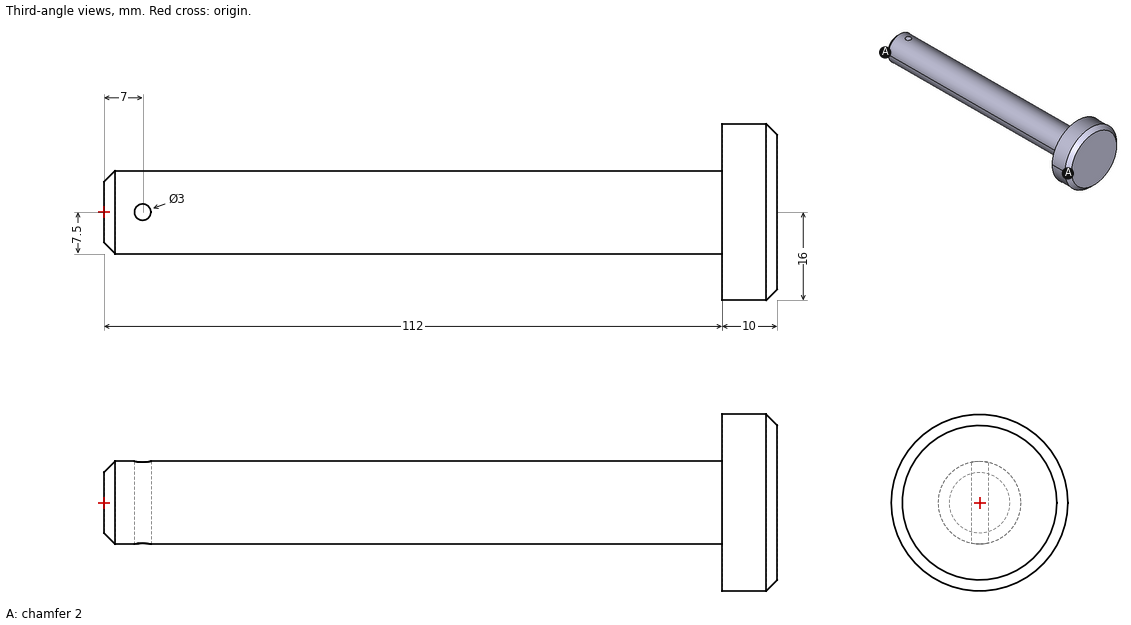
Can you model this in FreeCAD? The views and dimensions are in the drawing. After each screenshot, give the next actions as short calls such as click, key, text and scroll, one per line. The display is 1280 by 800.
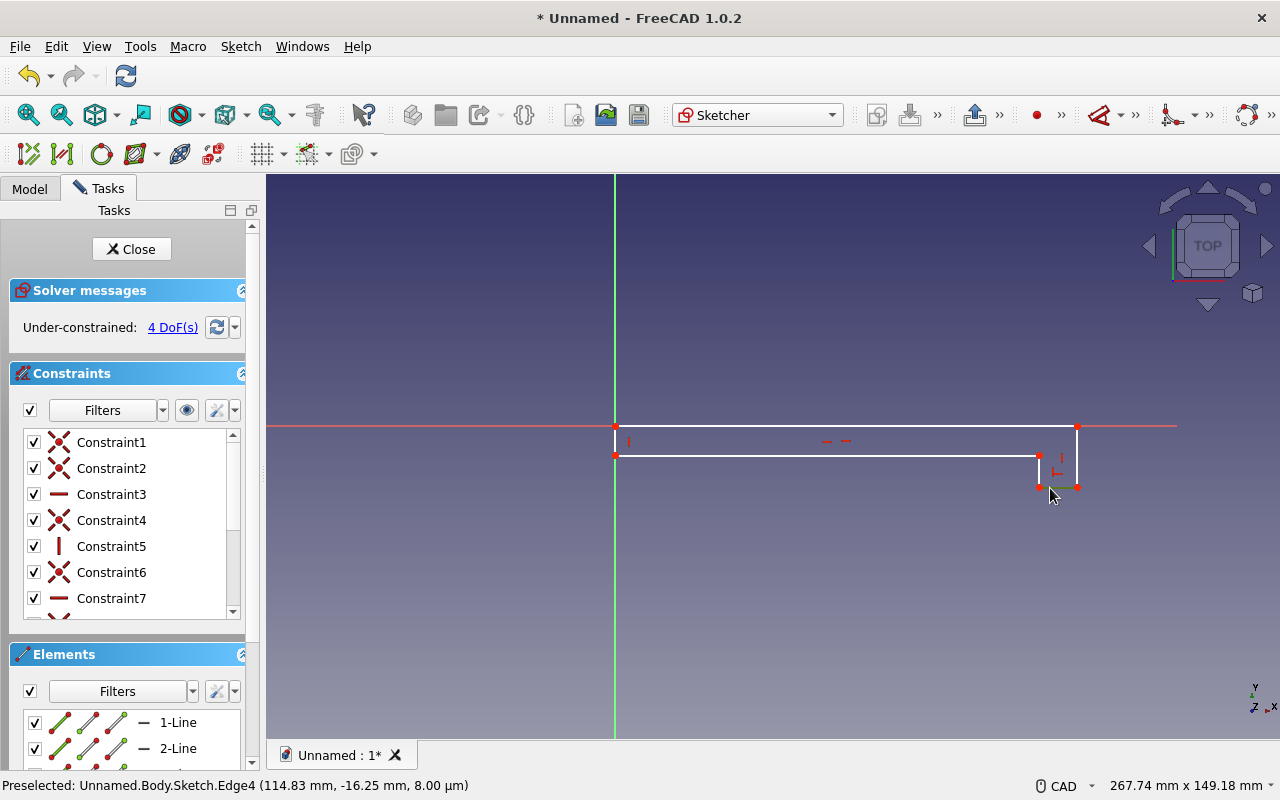
click(1120, 116)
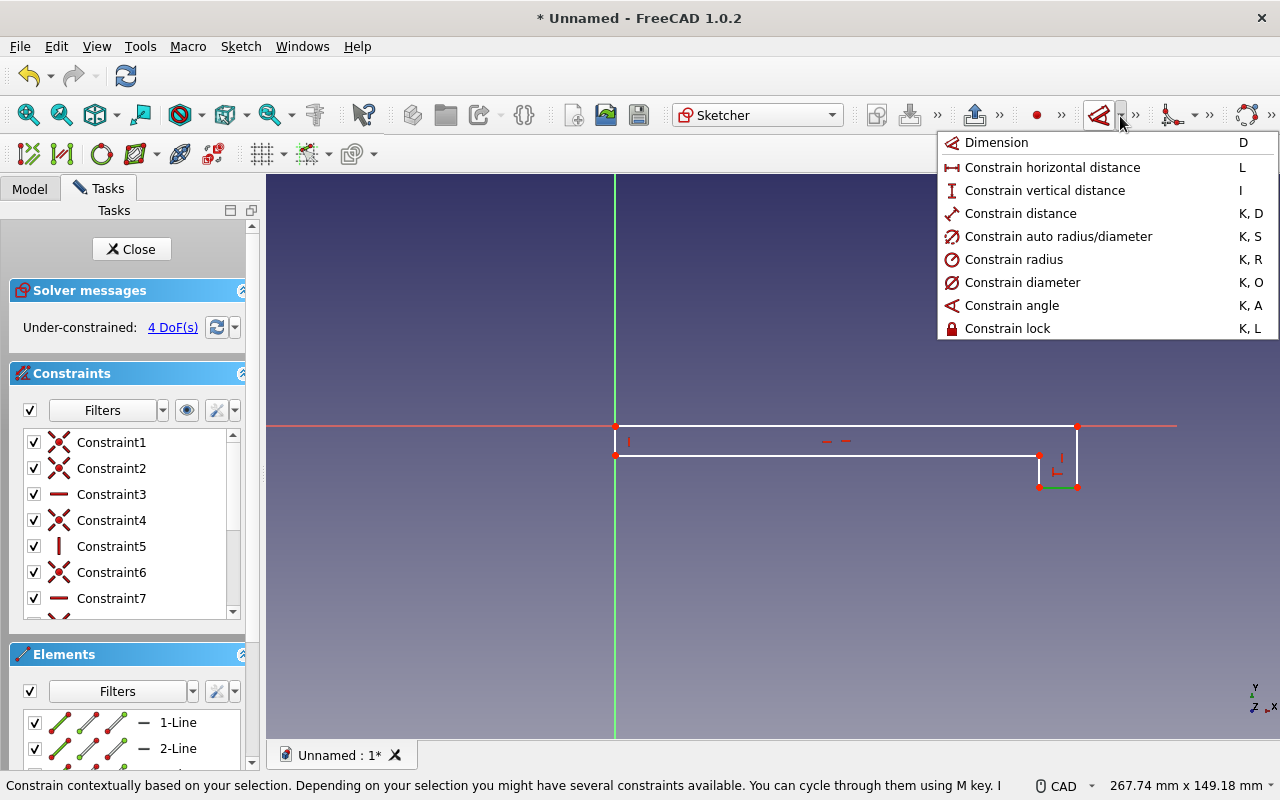
click(1108, 168)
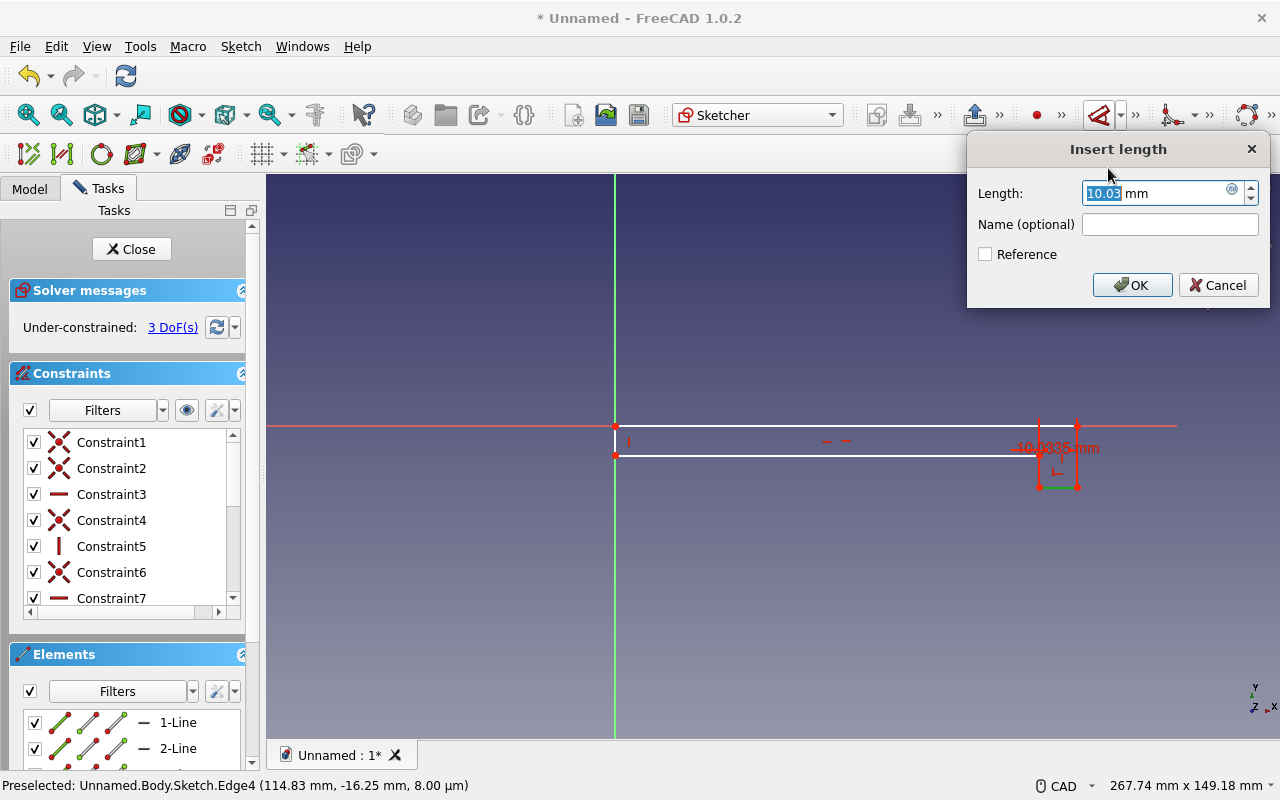
text(10)
key(Return)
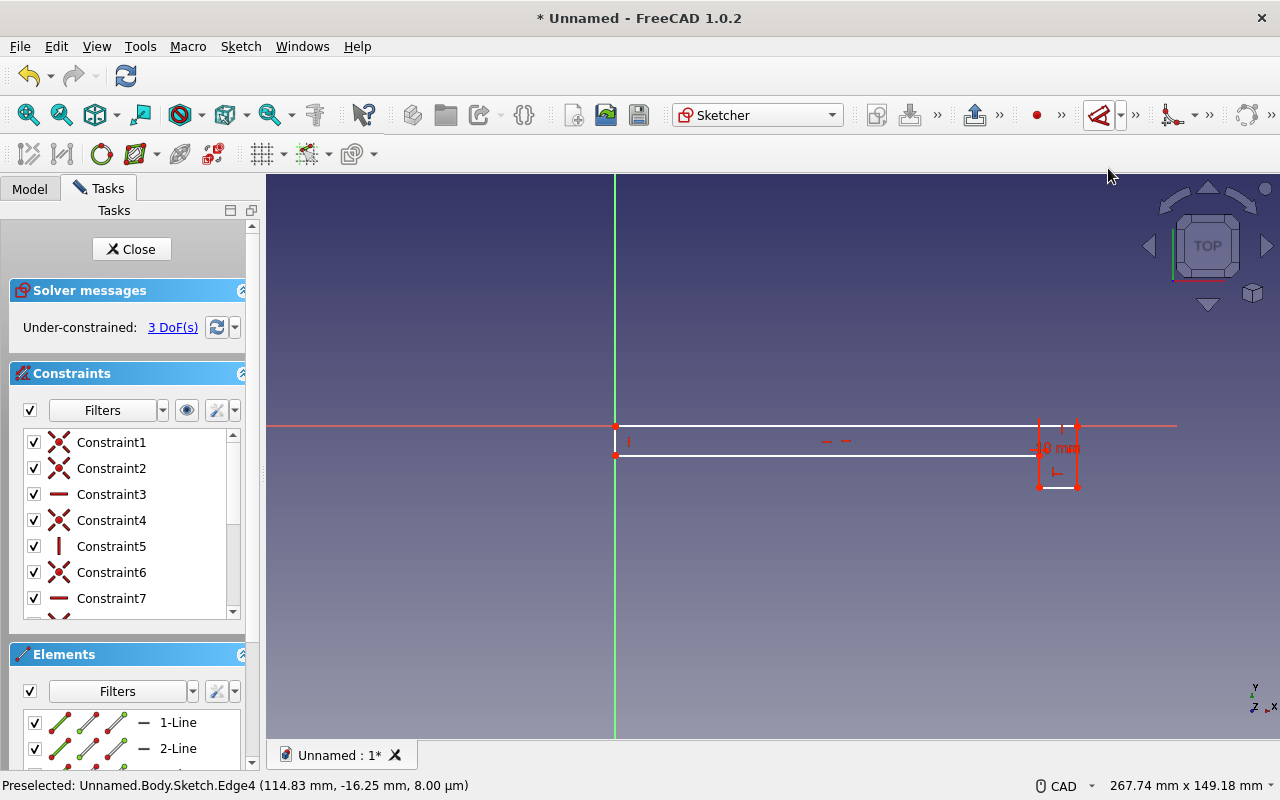
click(1077, 470)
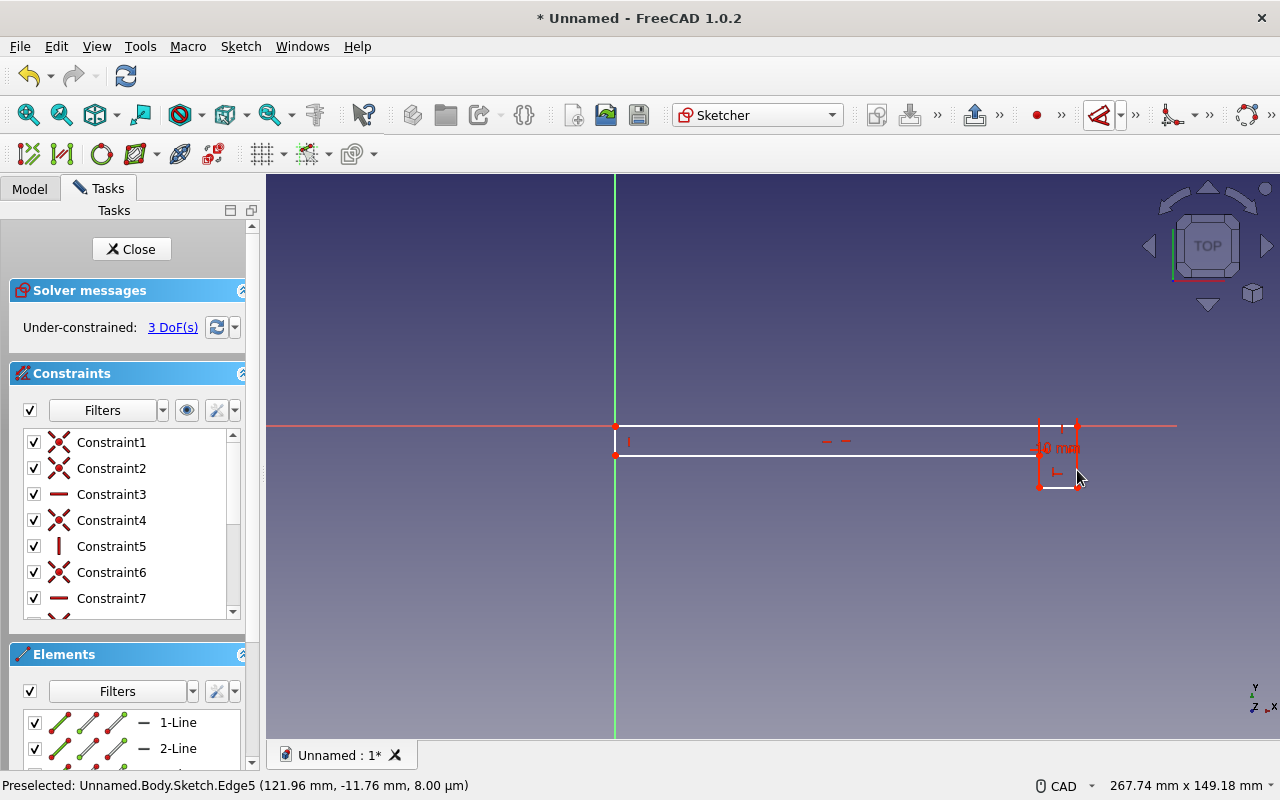
key(i)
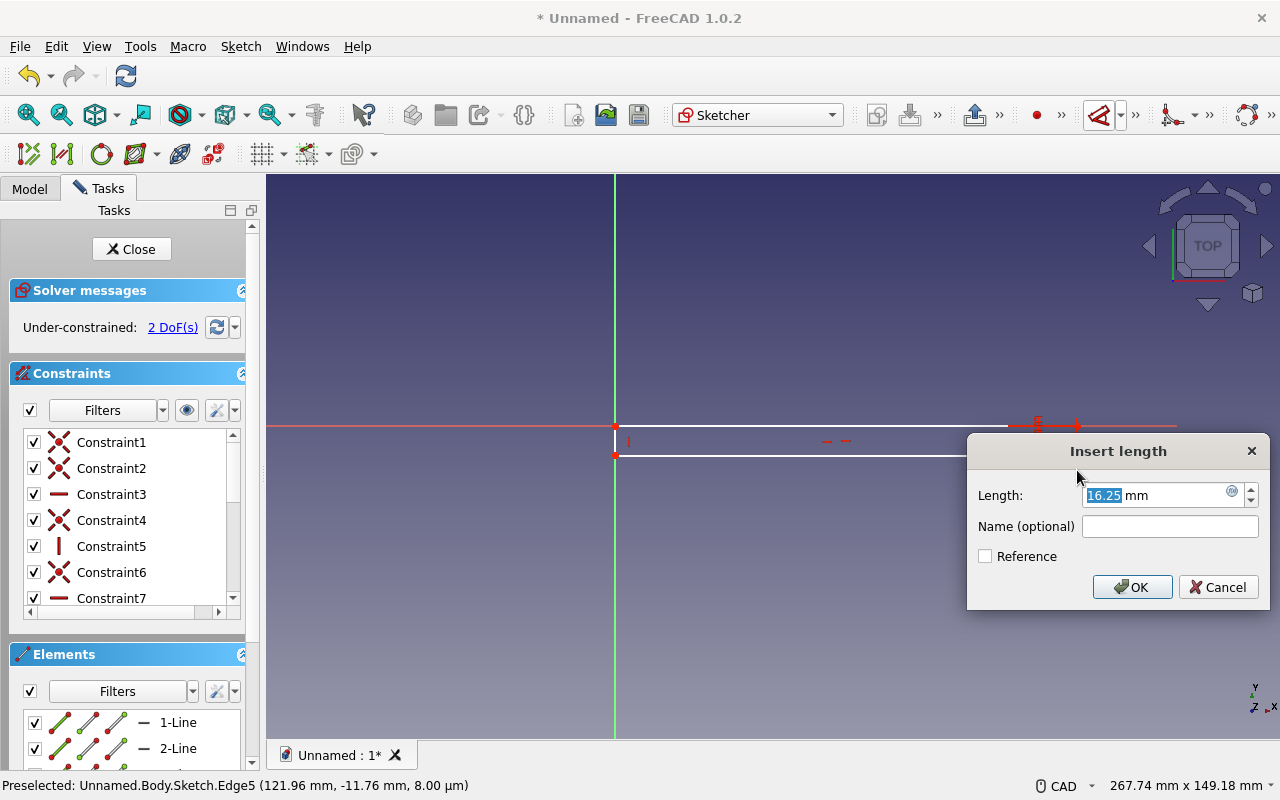
text(16)
key(Return)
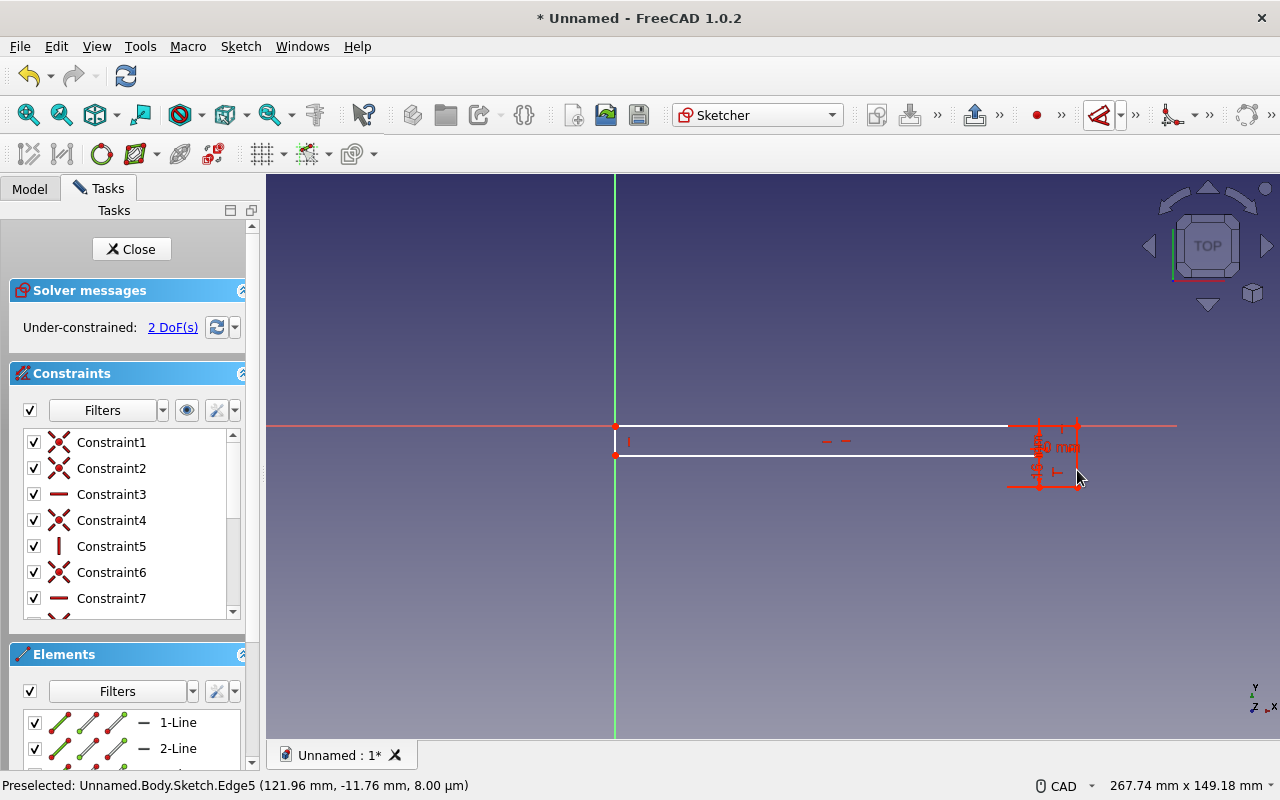
scroll(615, 438, up, 2)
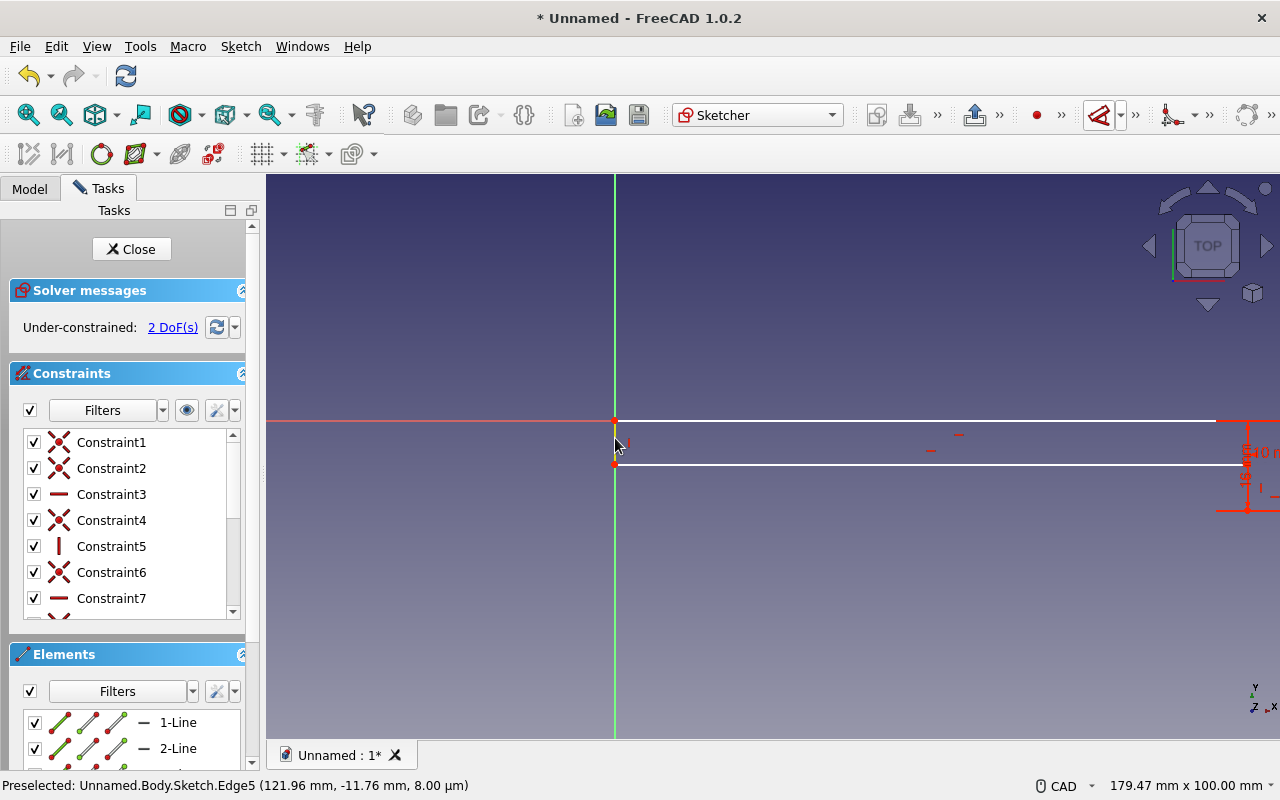
click(615, 438)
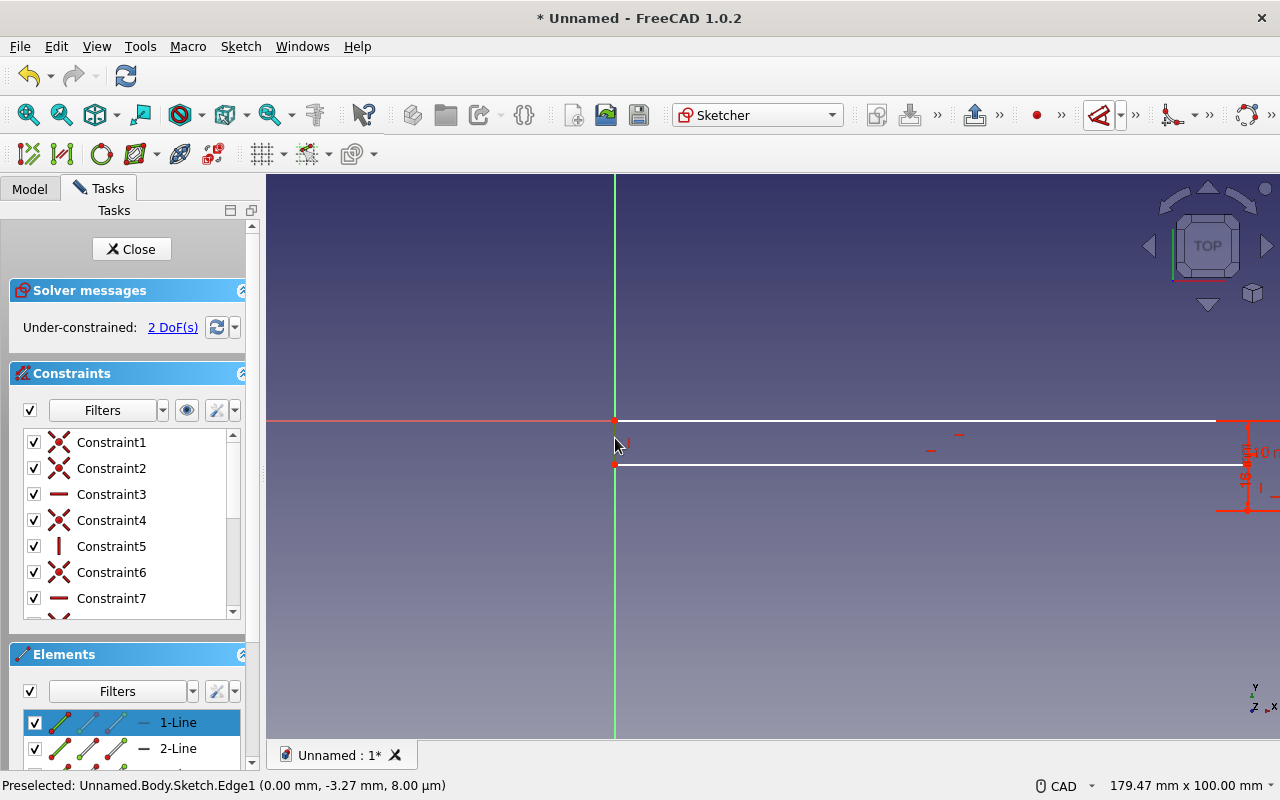
click(1120, 116)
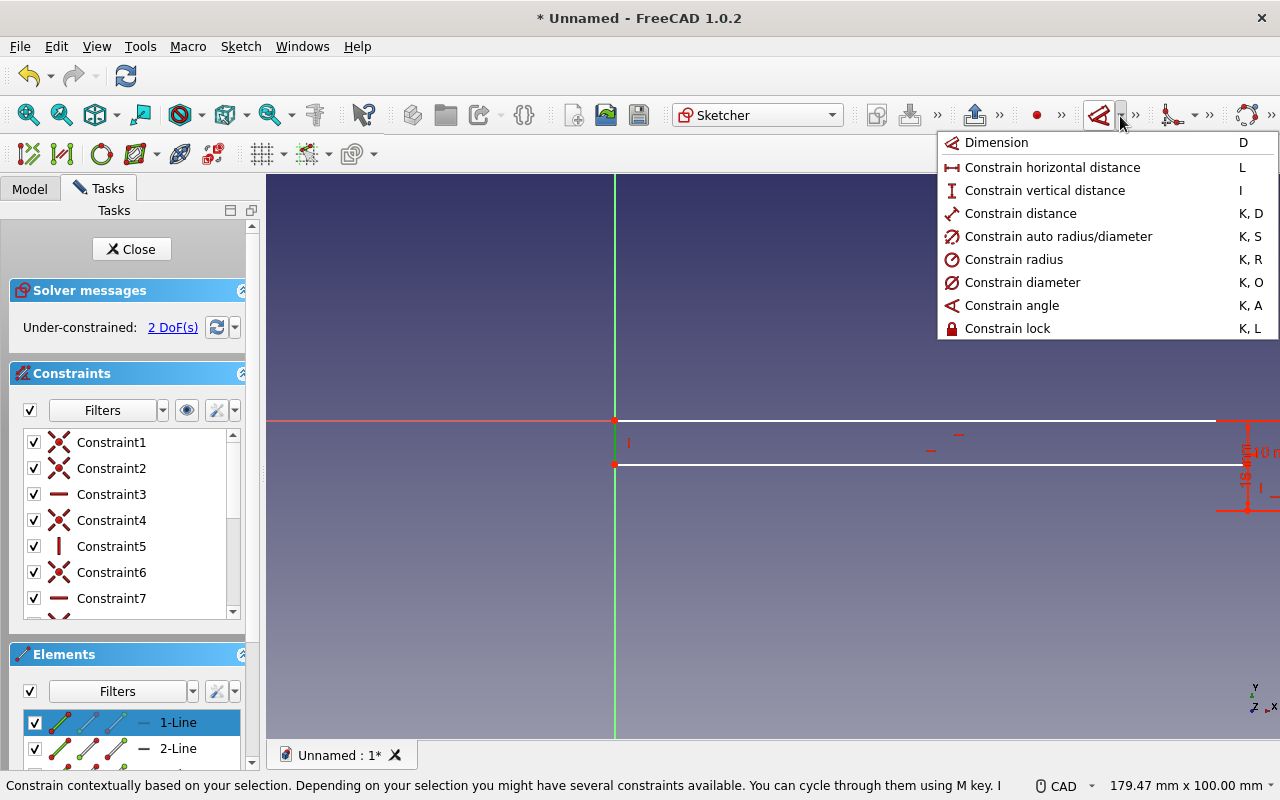
click(1108, 190)